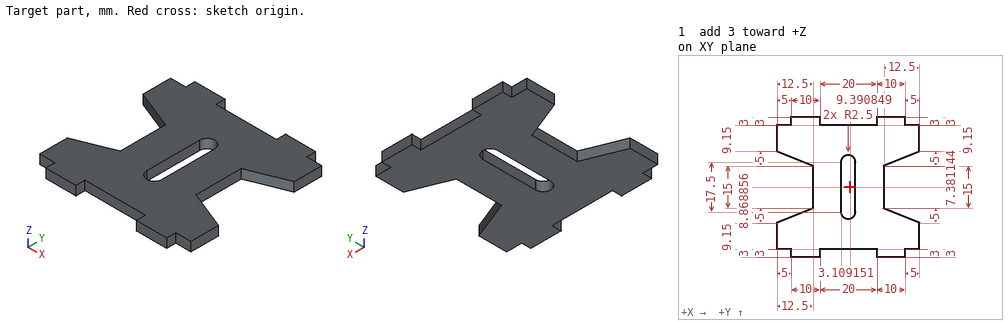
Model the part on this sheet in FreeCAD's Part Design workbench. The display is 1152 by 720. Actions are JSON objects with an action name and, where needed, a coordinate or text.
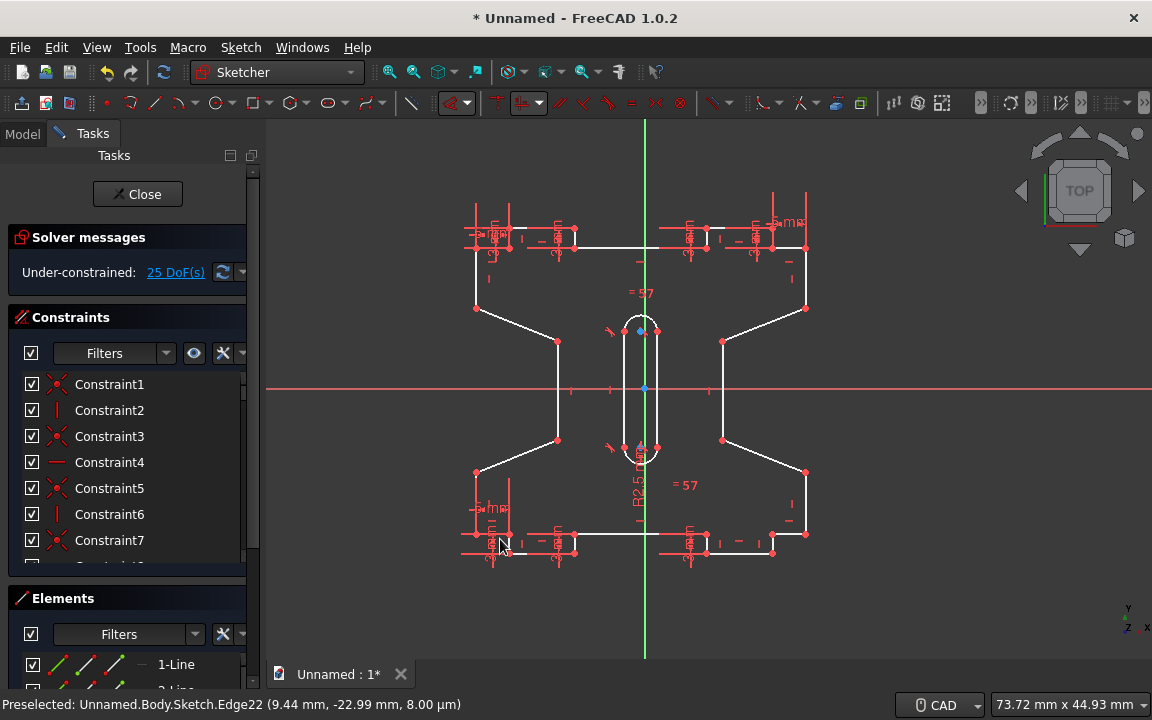
{"action": "scroll", "coordinate": [773, 548], "scroll_direction": "up", "scroll_amount": 5}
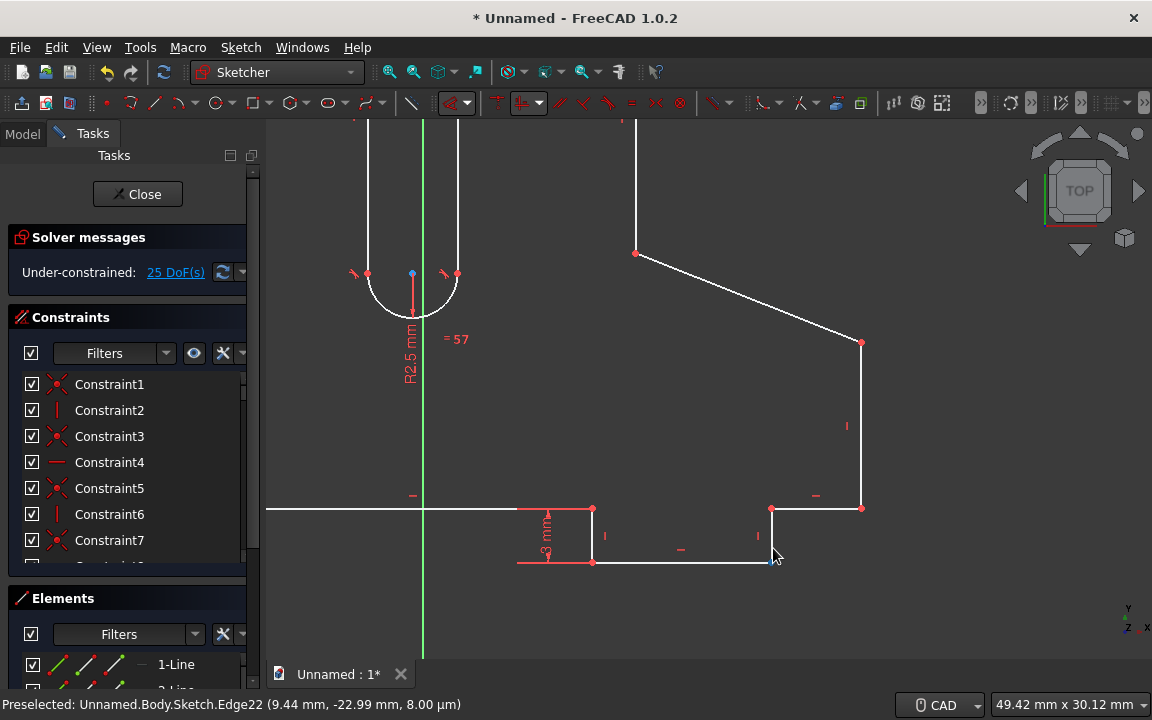
{"action": "left_click", "coordinate": [772, 546]}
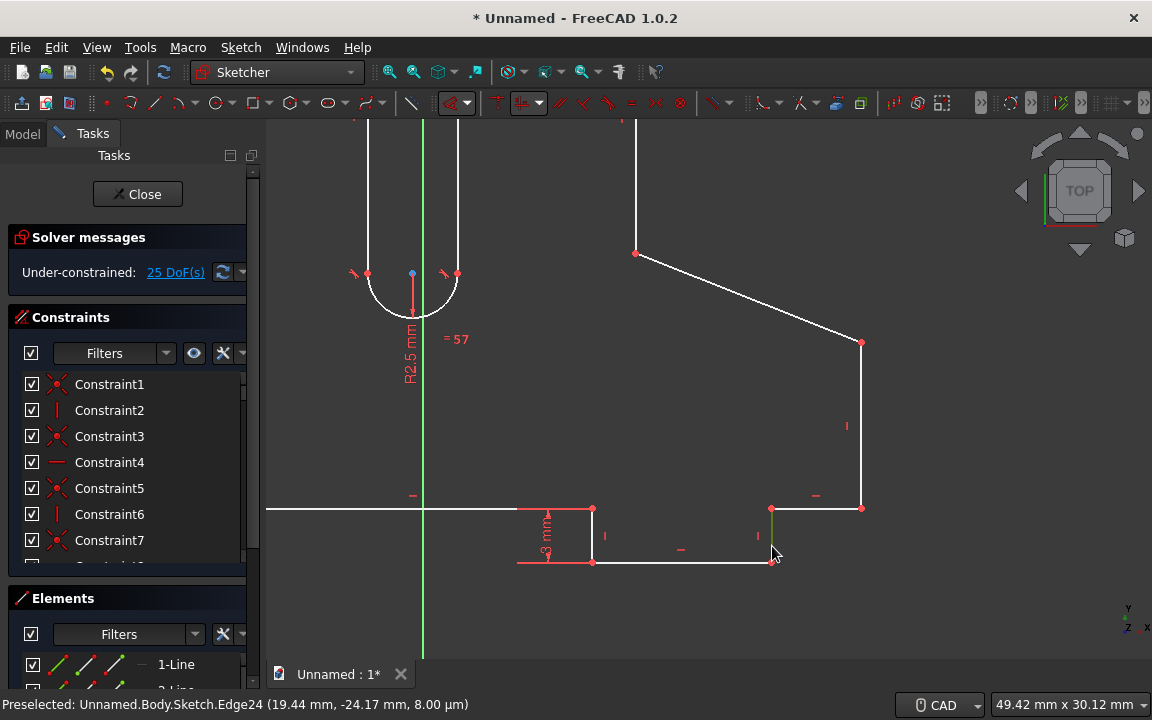
{"action": "left_click", "coordinate": [470, 104]}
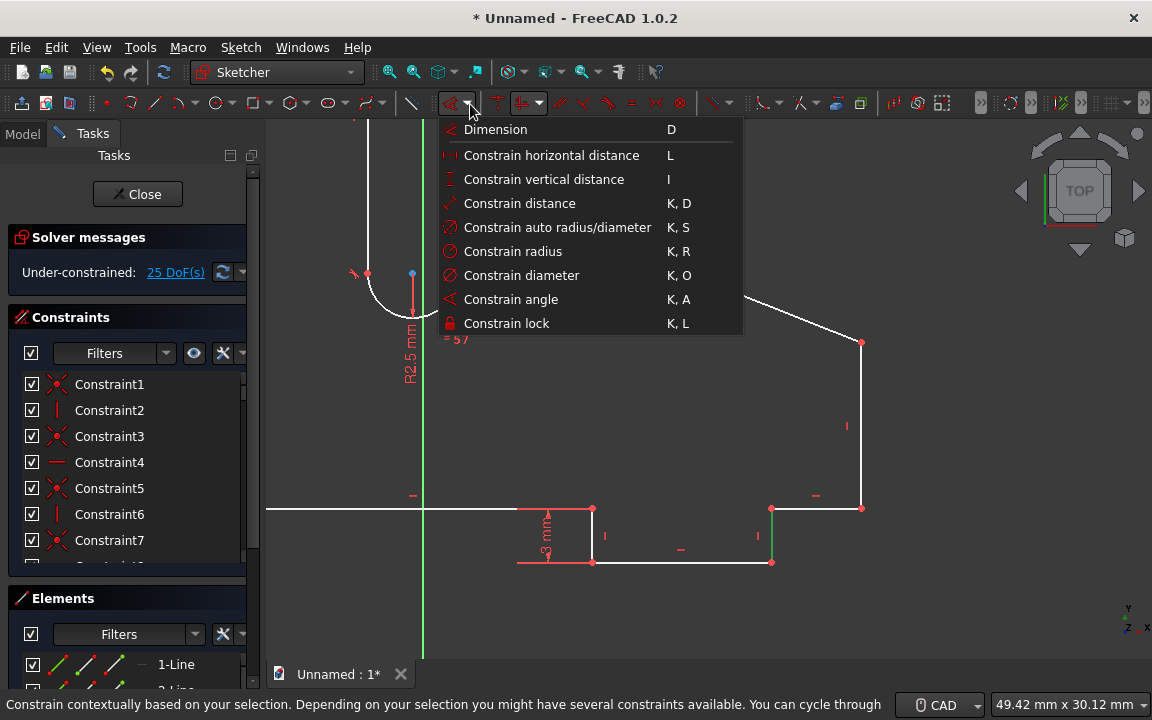
{"action": "left_click", "coordinate": [591, 179]}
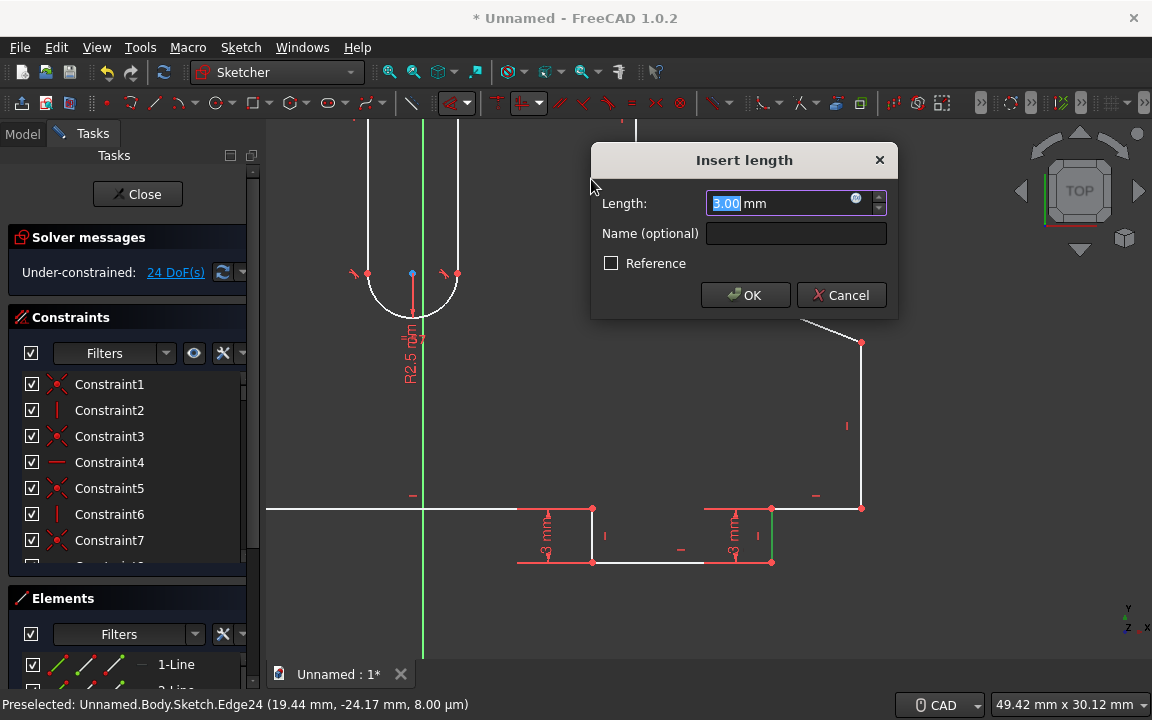
{"action": "type", "text": "3"}
{"action": "key", "text": "Return"}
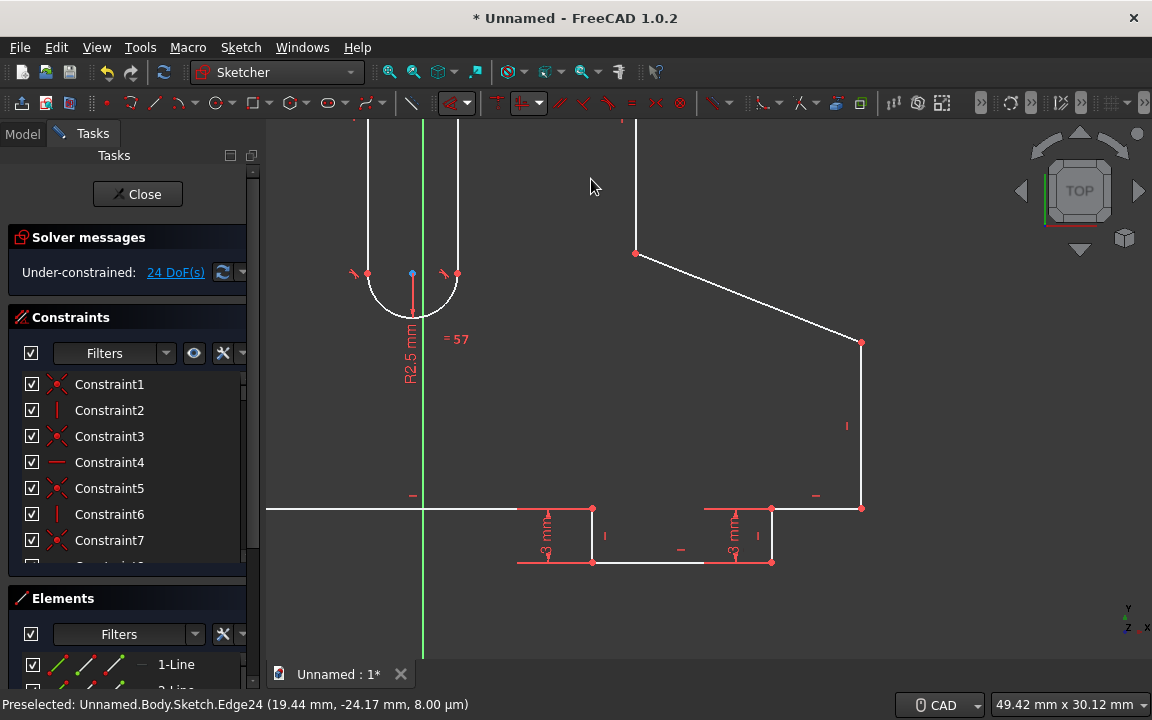
{"action": "left_click", "coordinate": [799, 509]}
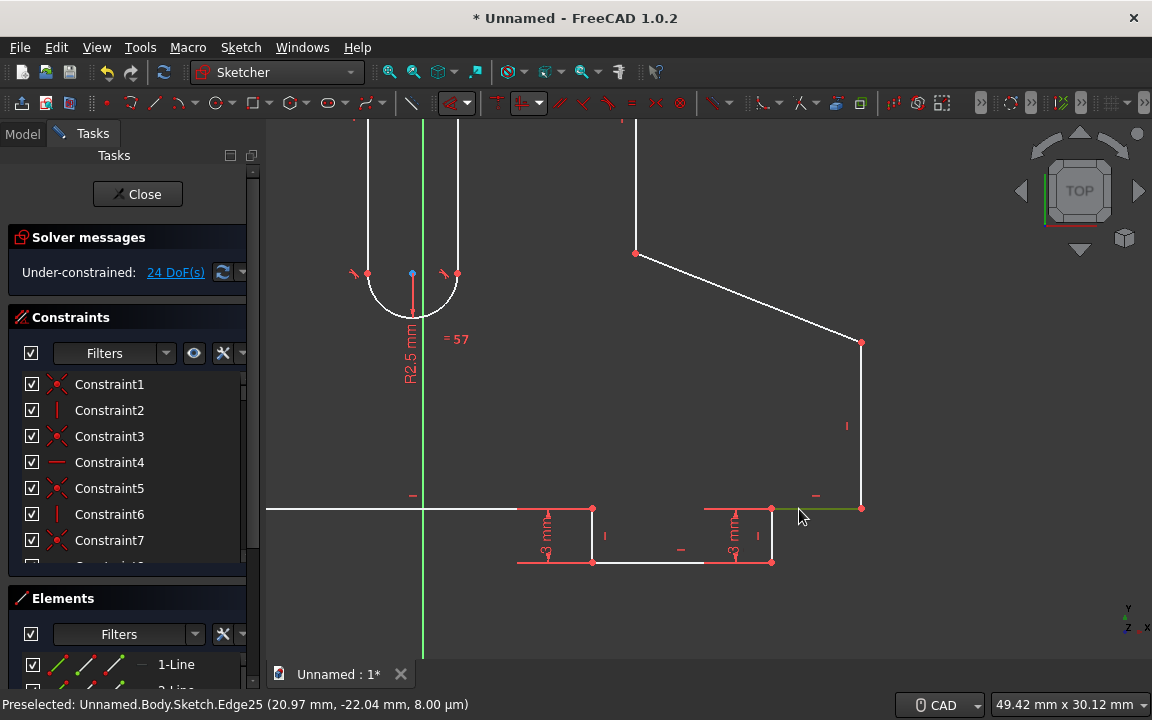
{"action": "left_click", "coordinate": [470, 104]}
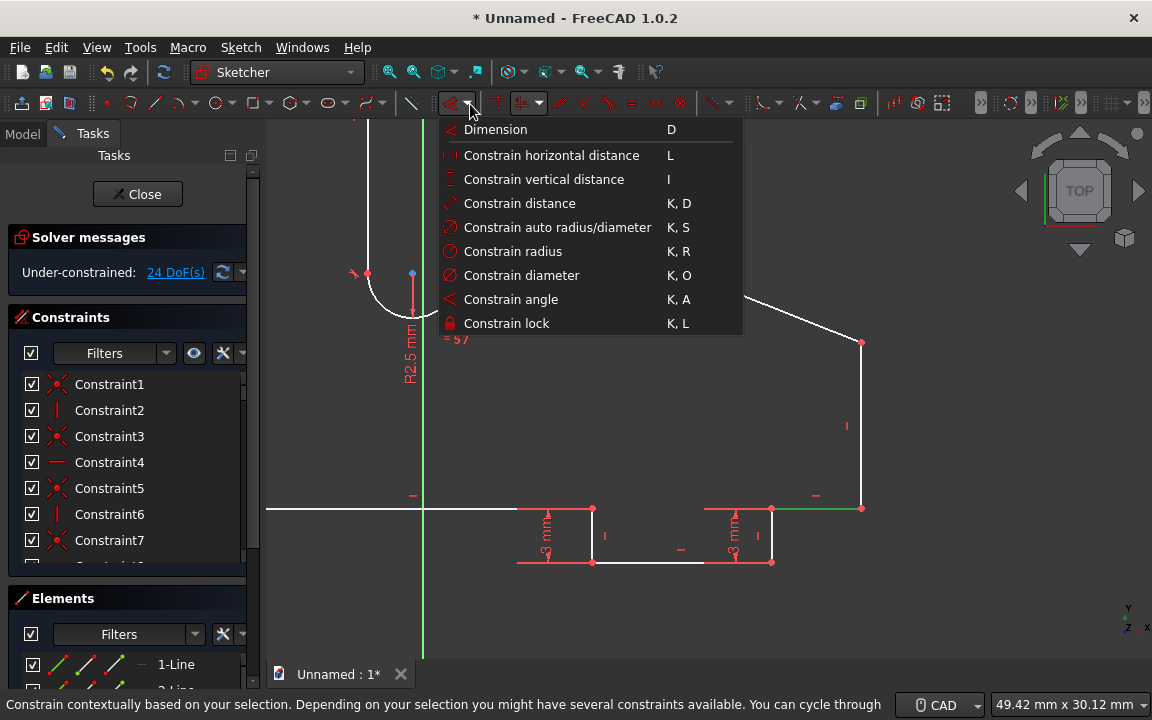
{"action": "left_click", "coordinate": [591, 155]}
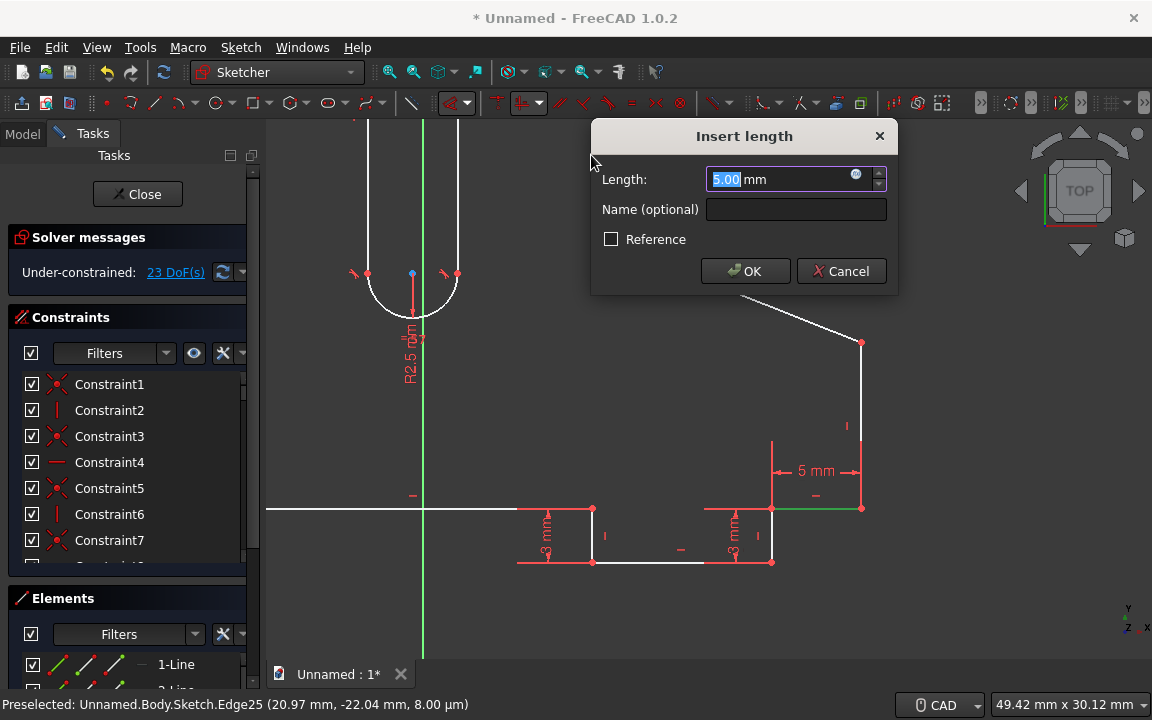
{"action": "type", "text": "5"}
{"action": "key", "text": "Return"}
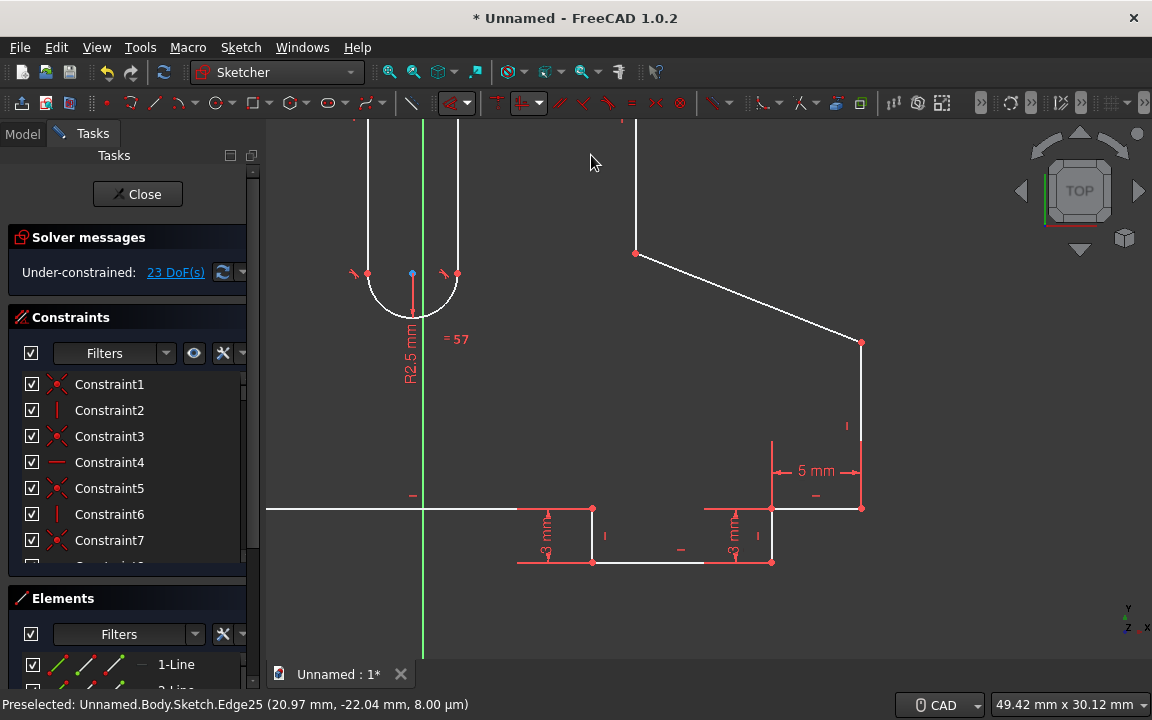
{"action": "scroll", "coordinate": [773, 548], "scroll_direction": "down", "scroll_amount": 5}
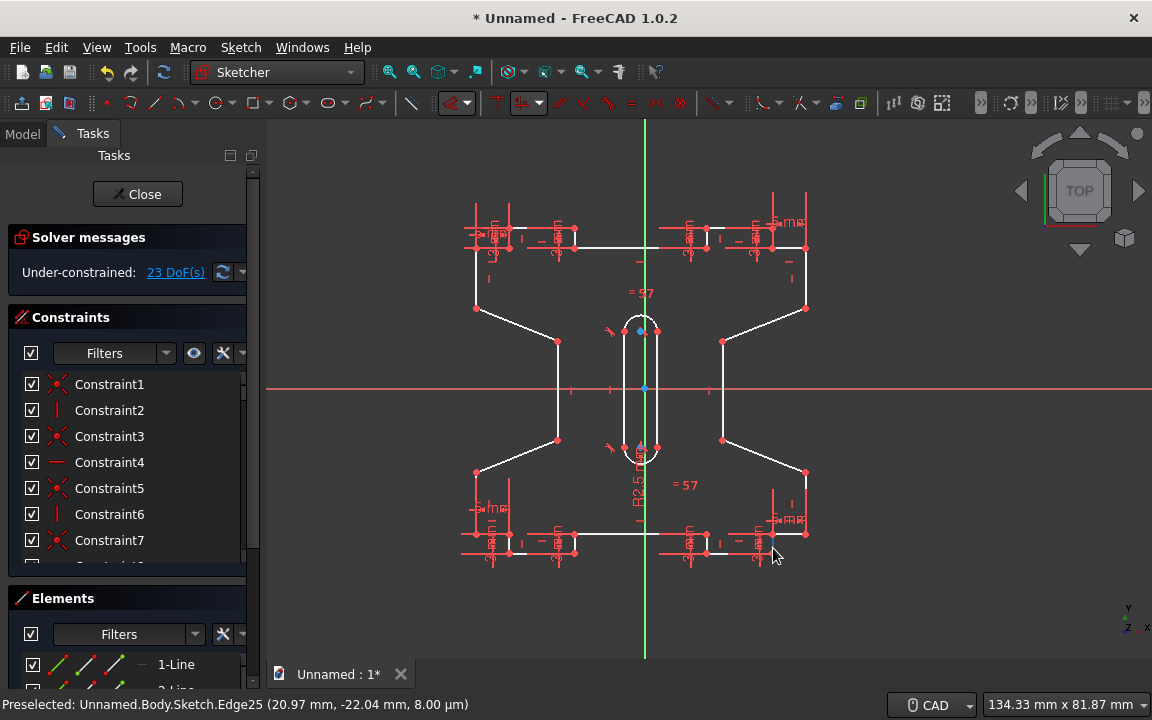
{"action": "left_click", "coordinate": [727, 228]}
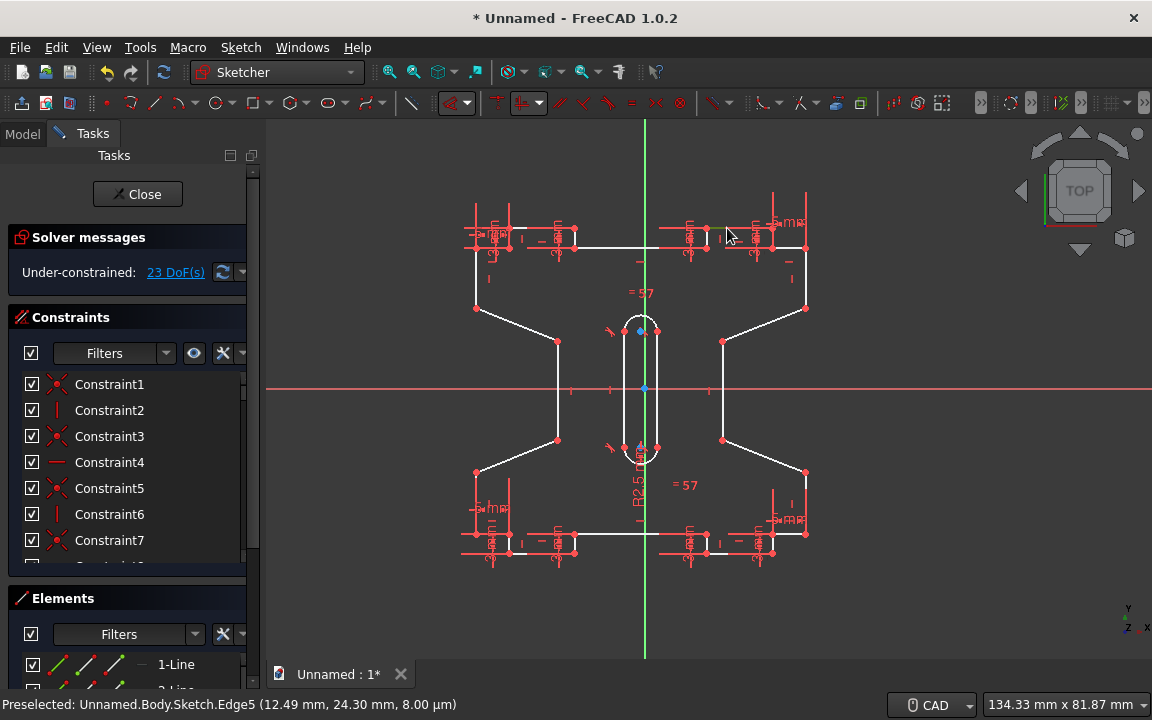
{"action": "left_click", "coordinate": [470, 104]}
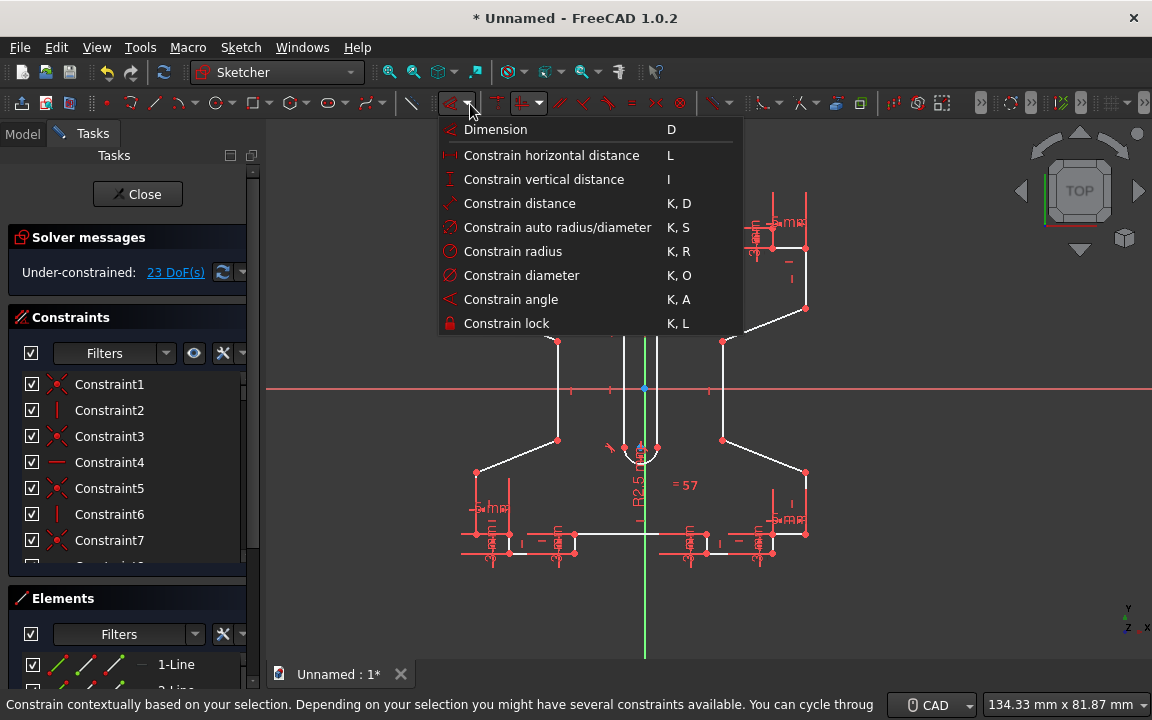
{"action": "left_click", "coordinate": [591, 155]}